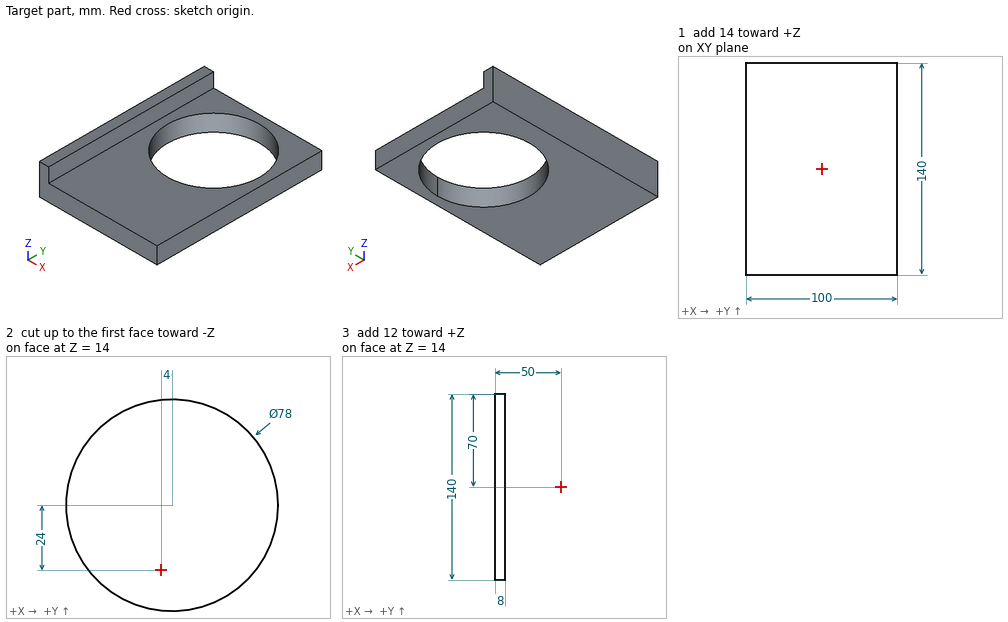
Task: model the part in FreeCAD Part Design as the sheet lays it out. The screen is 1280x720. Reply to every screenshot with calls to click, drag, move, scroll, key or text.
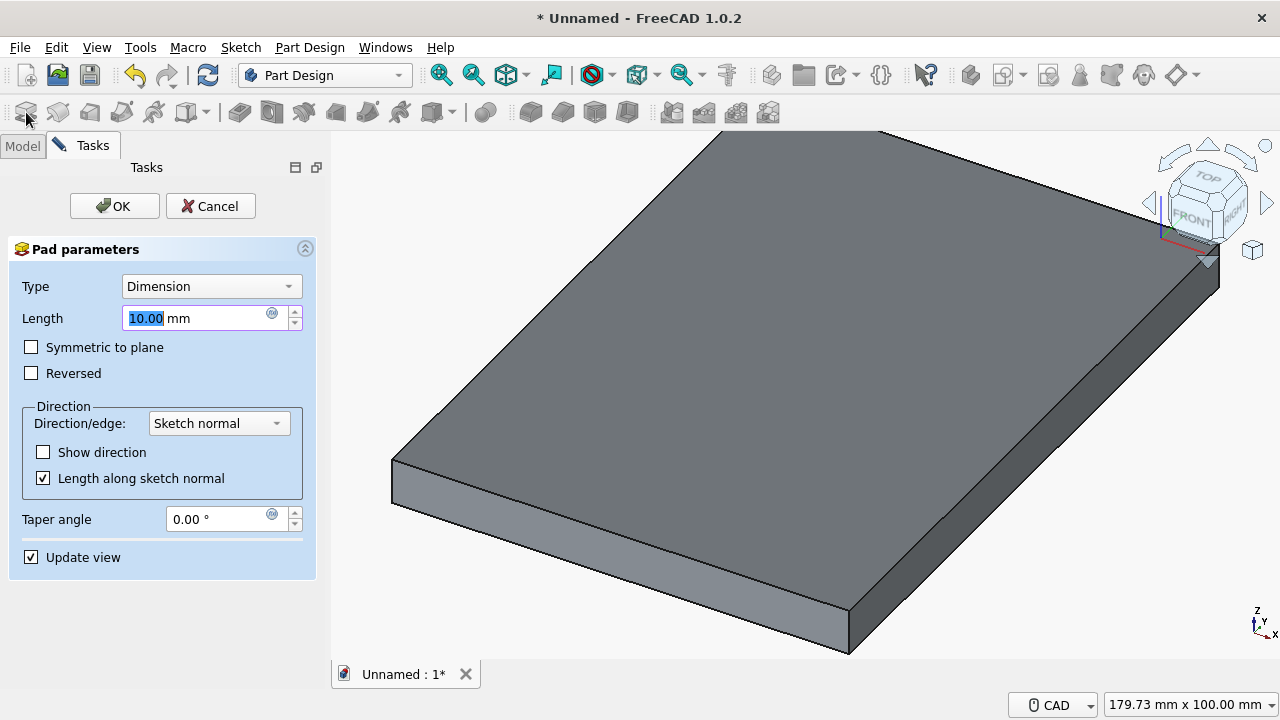
text(14)
key(Tab)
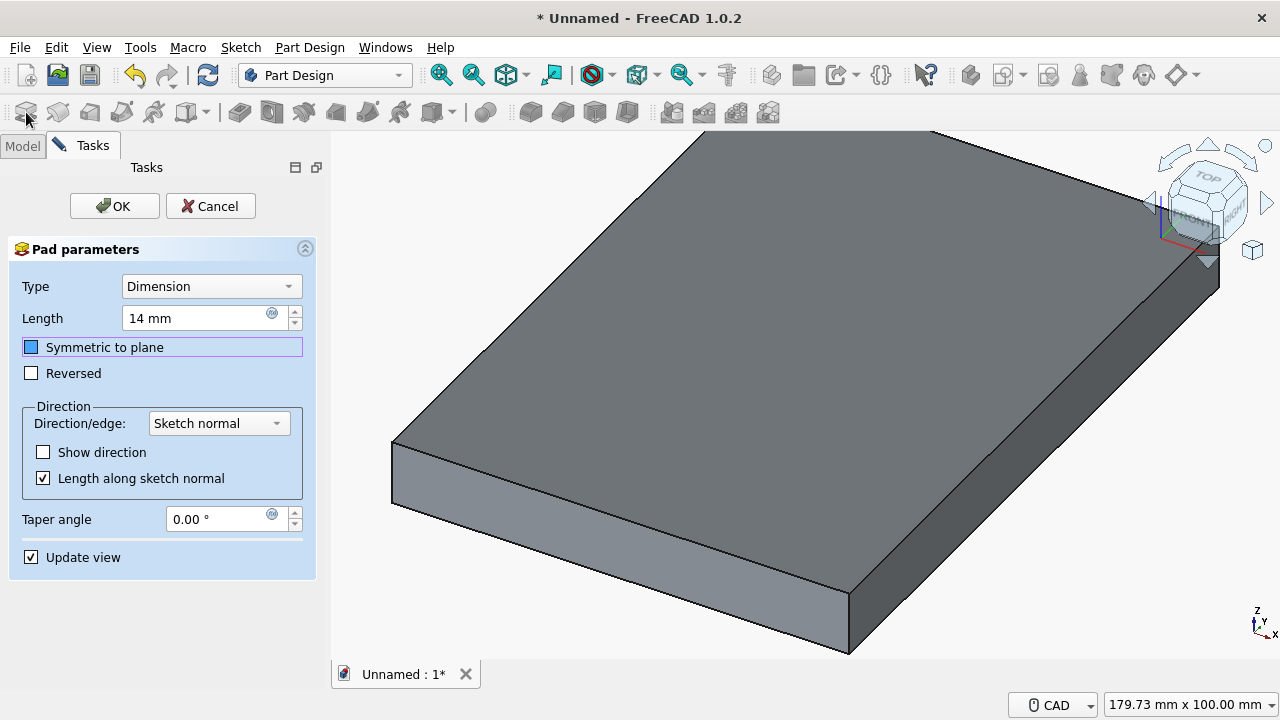
click(115, 206)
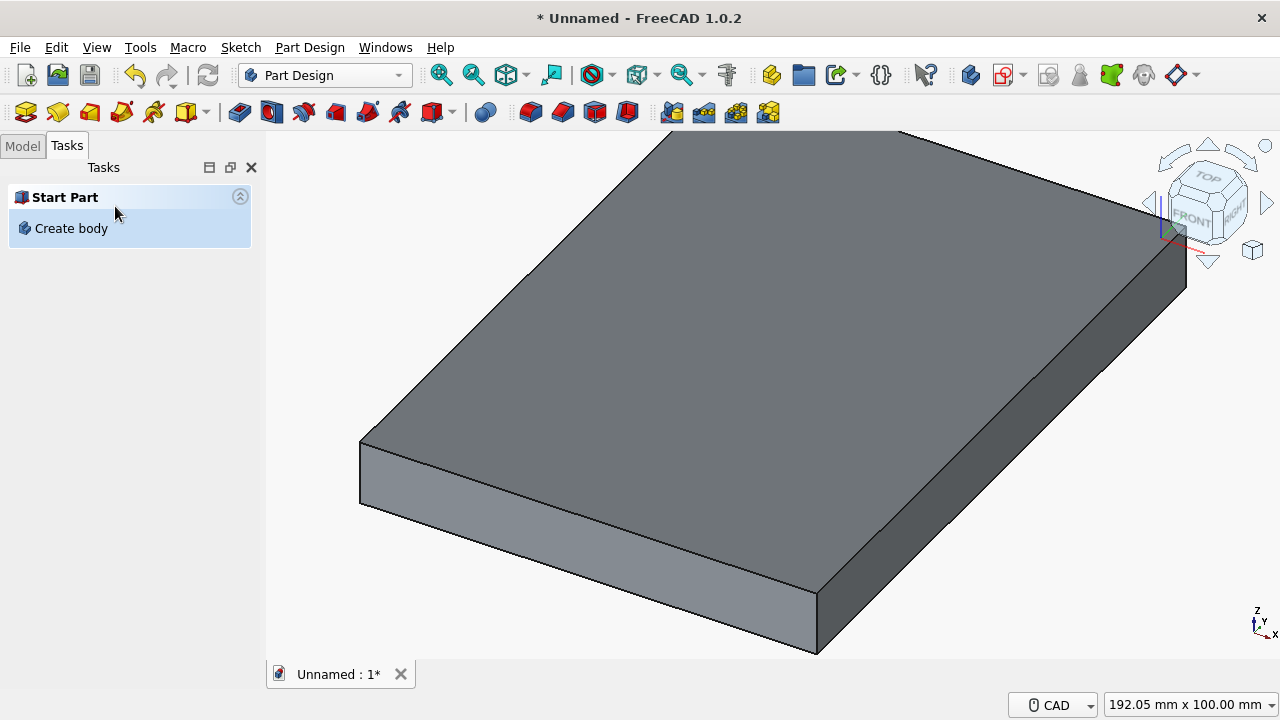
click(442, 76)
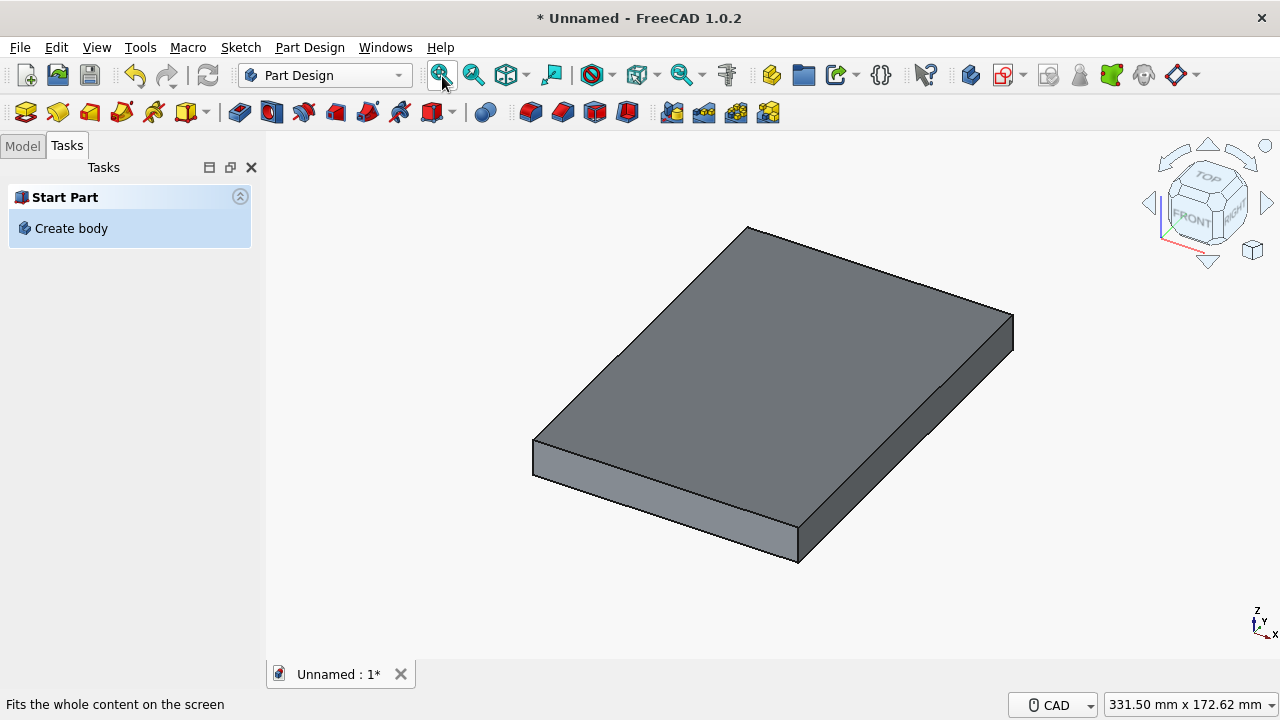
click(804, 346)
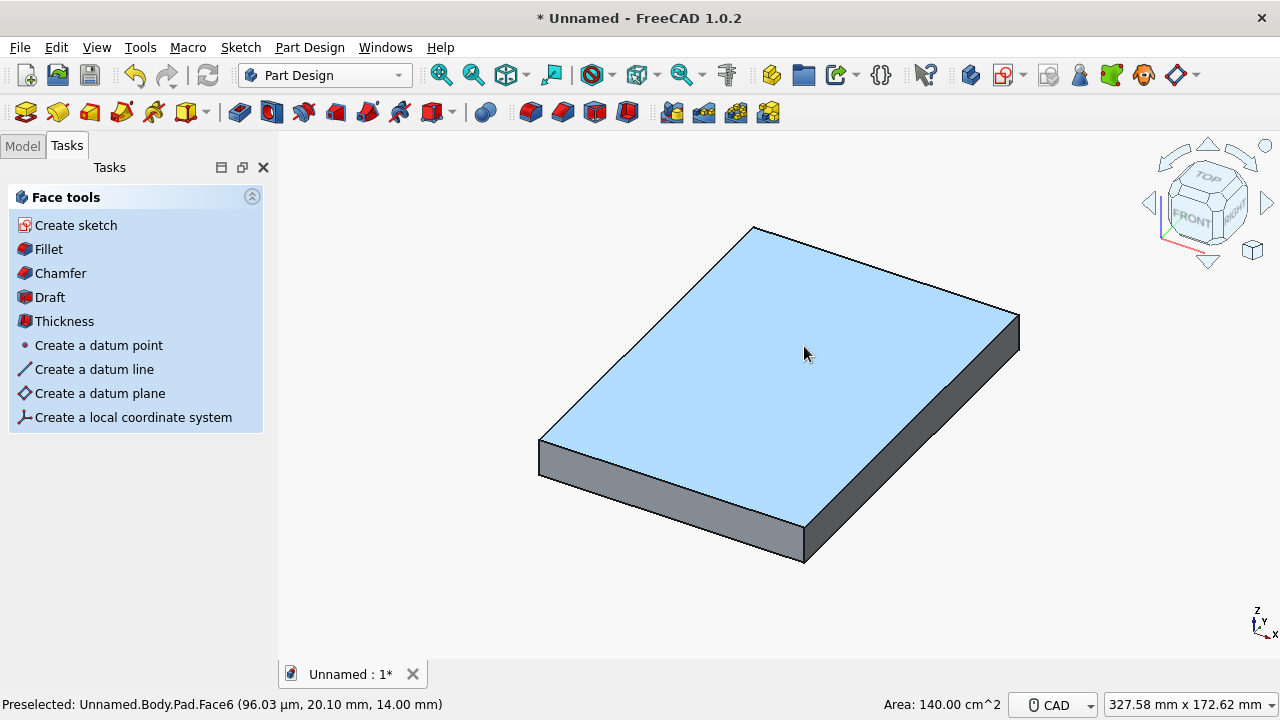
click(1004, 76)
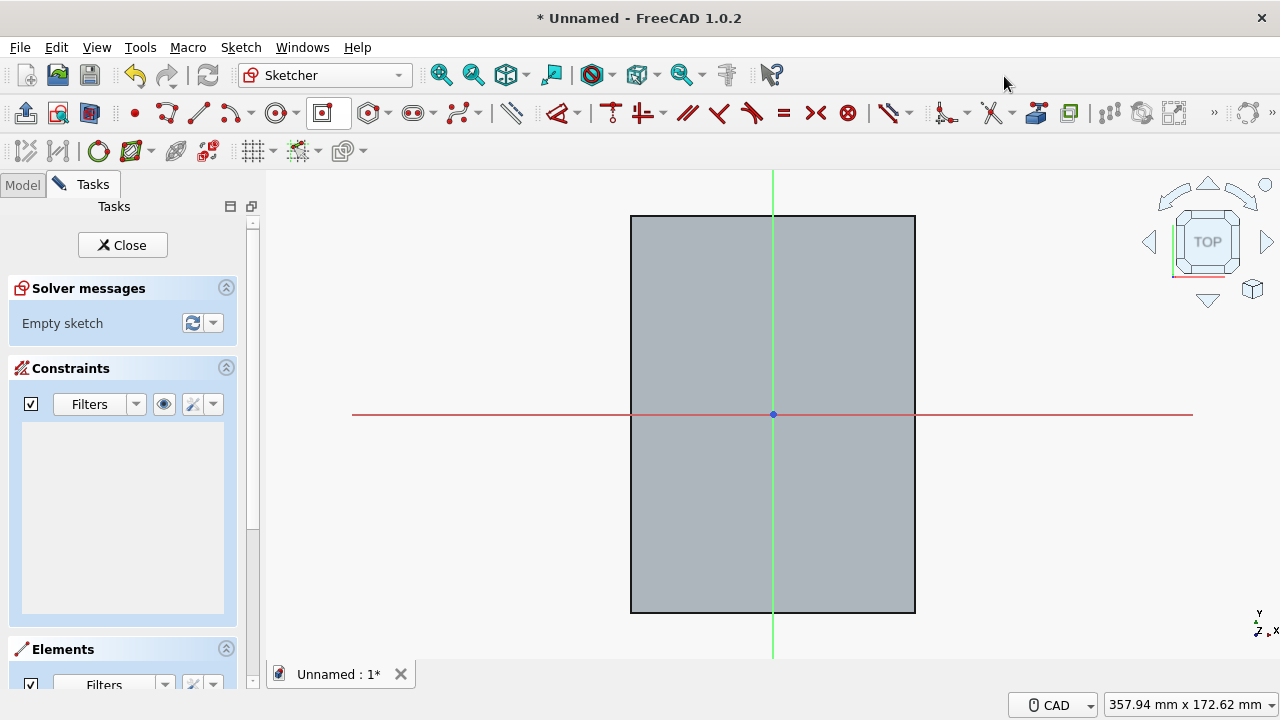
scroll(947, 208, up, 2)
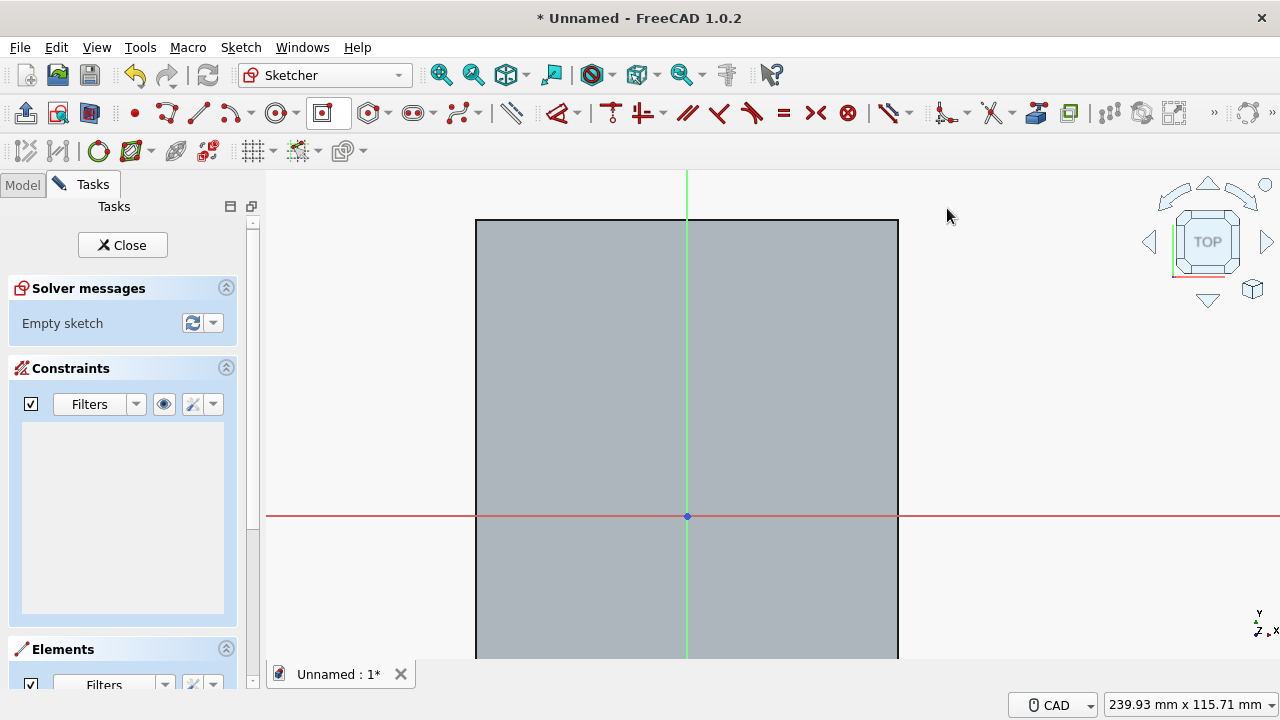
key(g)
key(c)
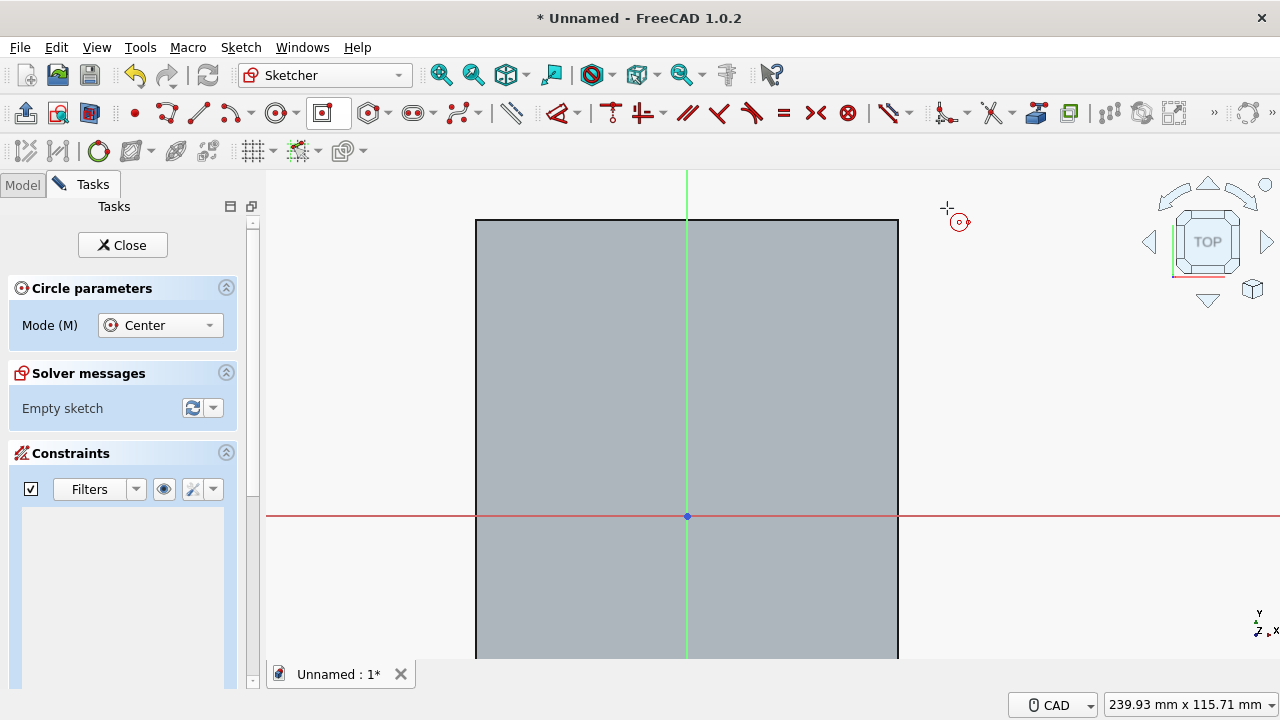
click(704, 415)
move(821, 298)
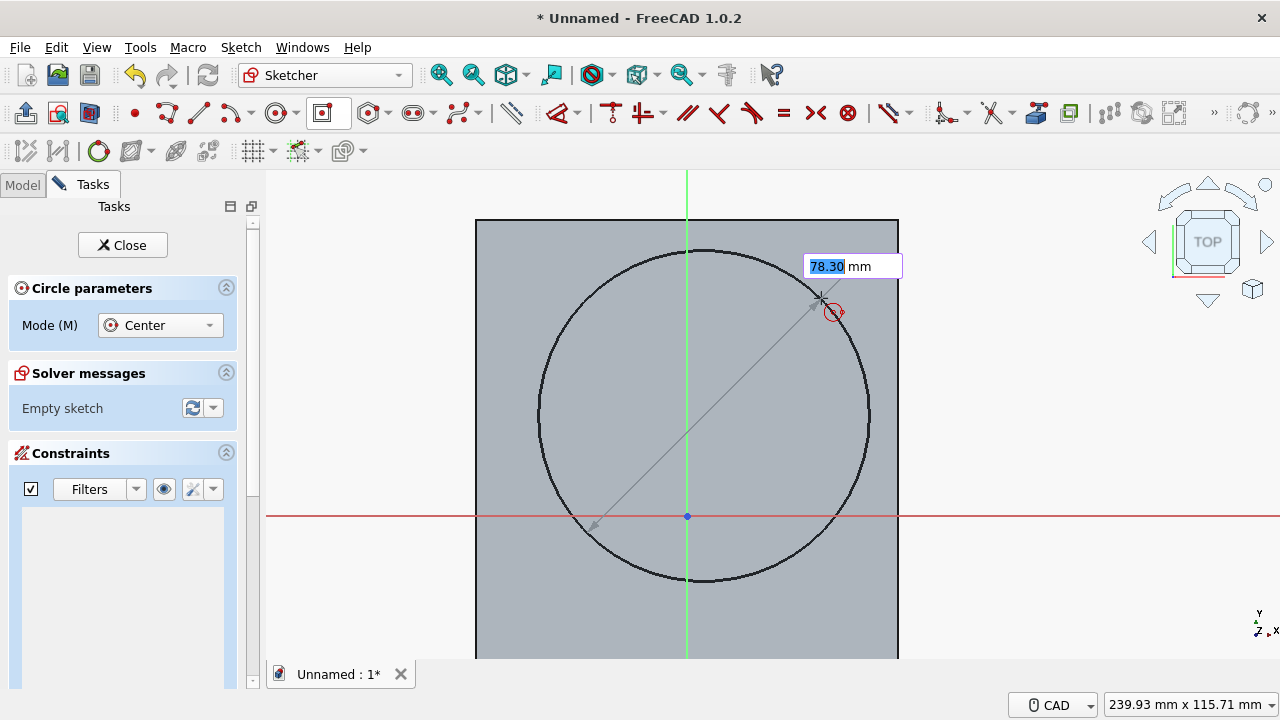
text(78)
key(Return)
key(Escape)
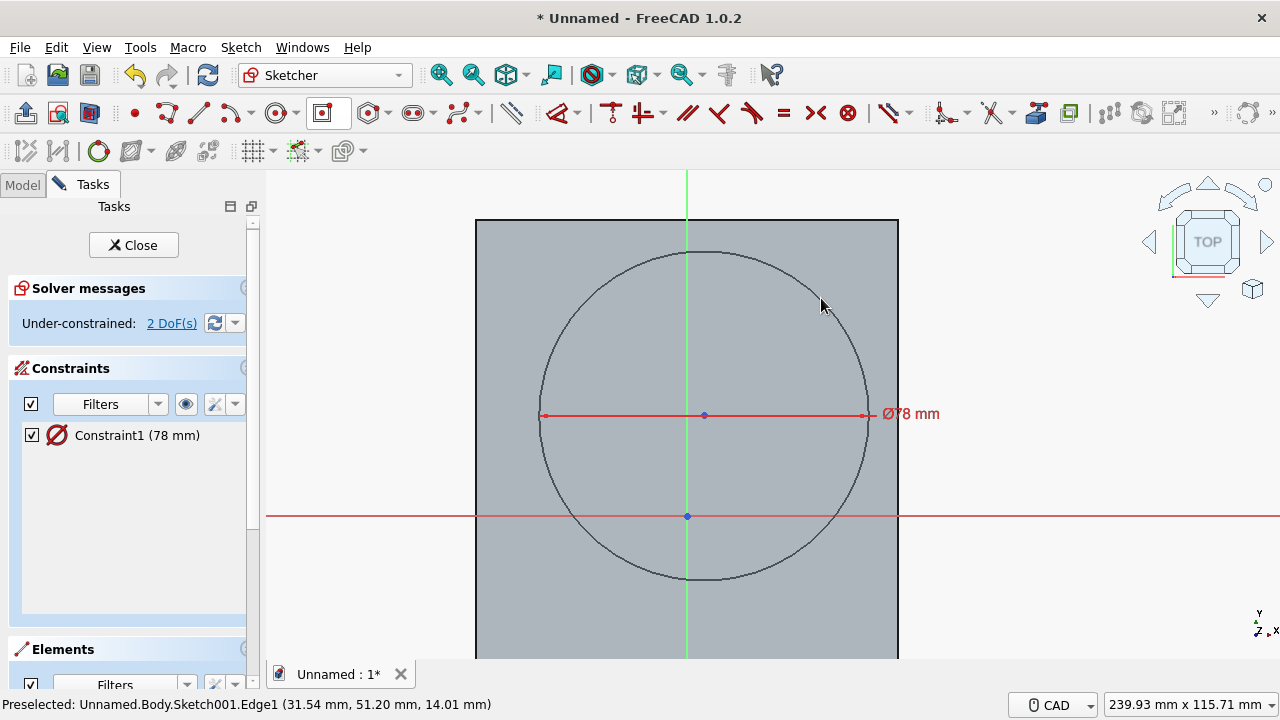
scroll(704, 416, up, 5)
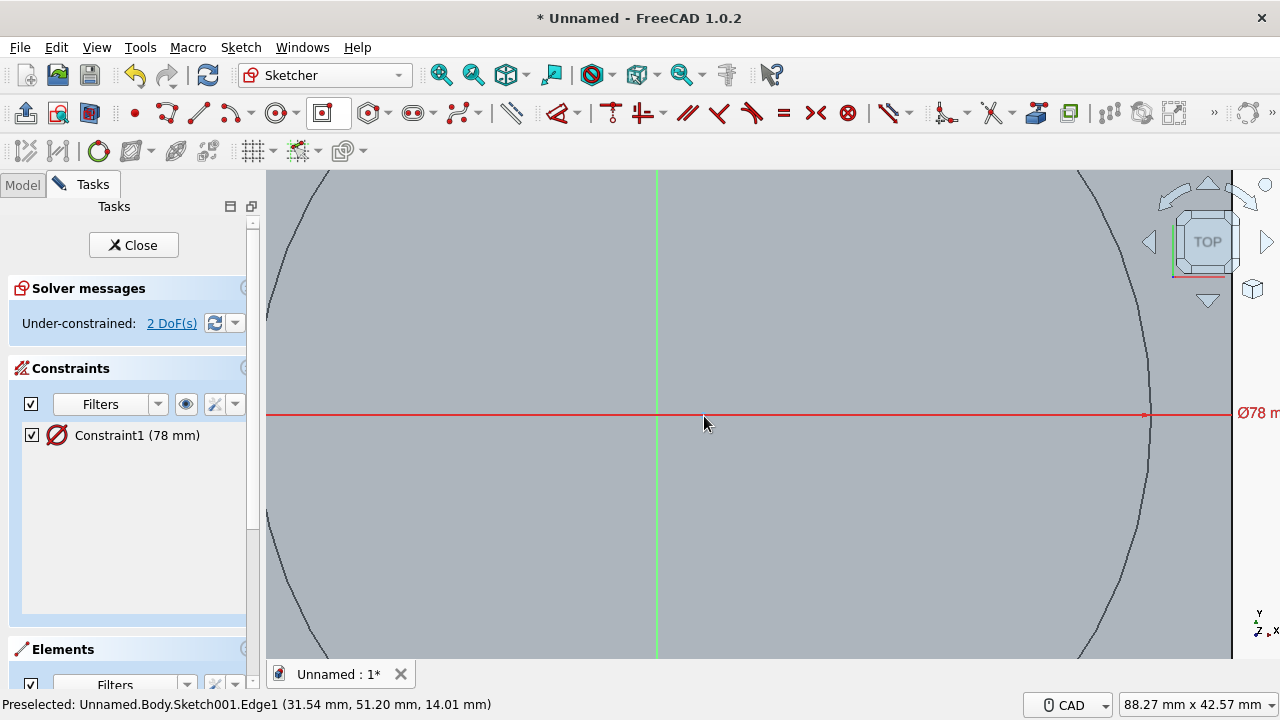
click(703, 415)